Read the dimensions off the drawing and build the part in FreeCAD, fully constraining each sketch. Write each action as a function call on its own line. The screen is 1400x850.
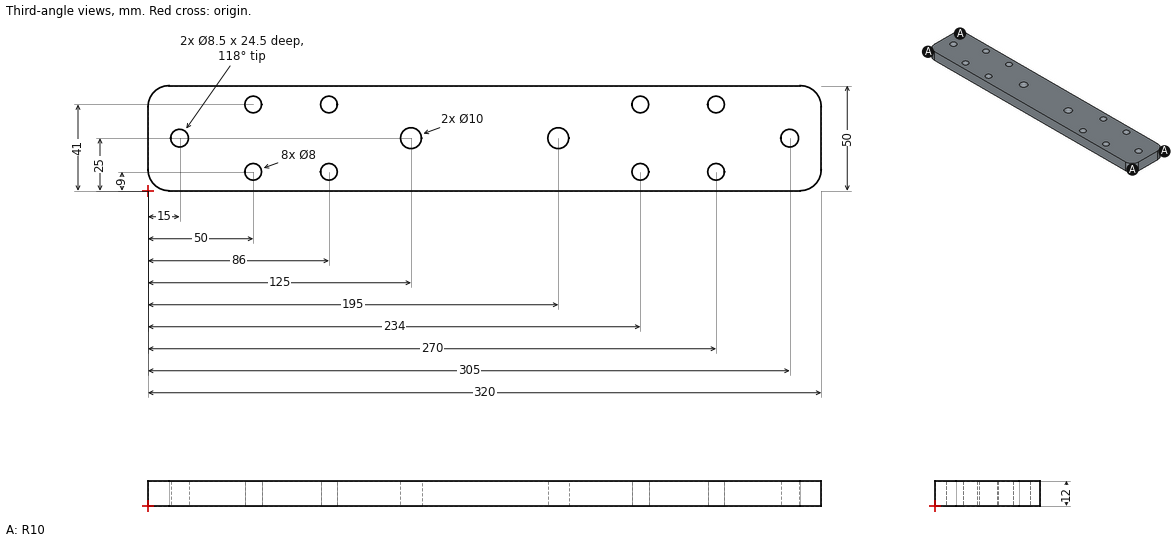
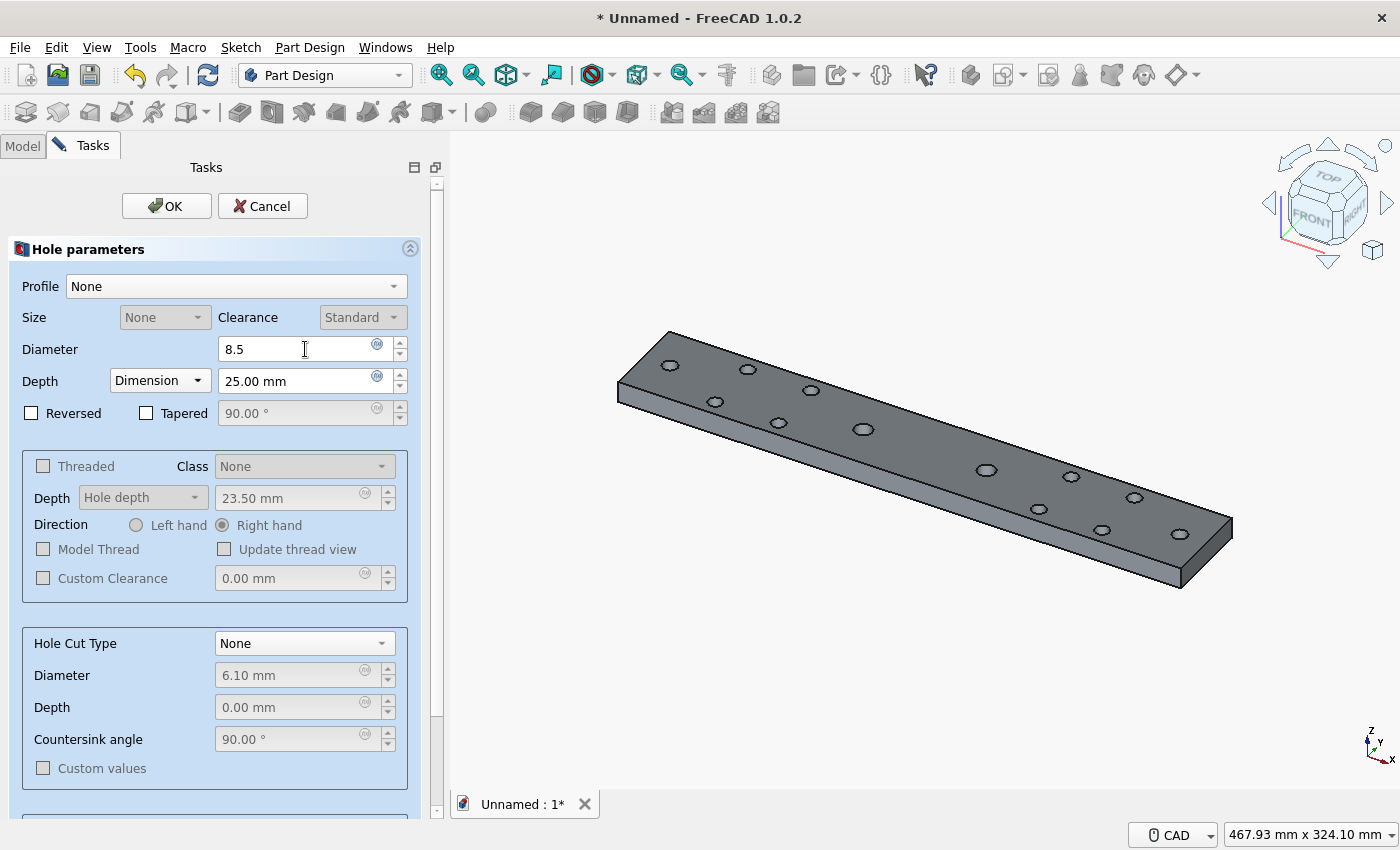
triple_click(305, 381)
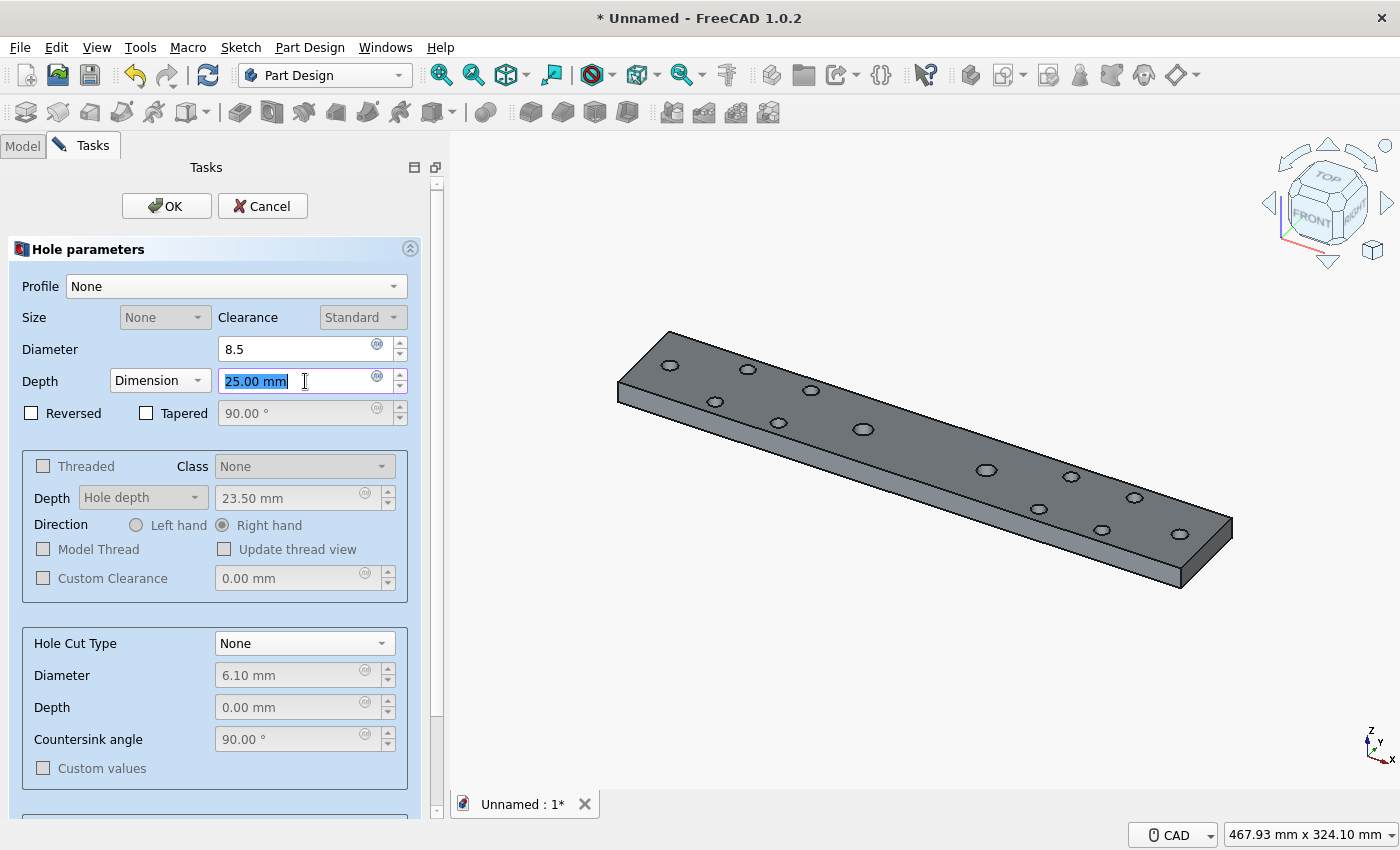
text(24.5)
key(Tab)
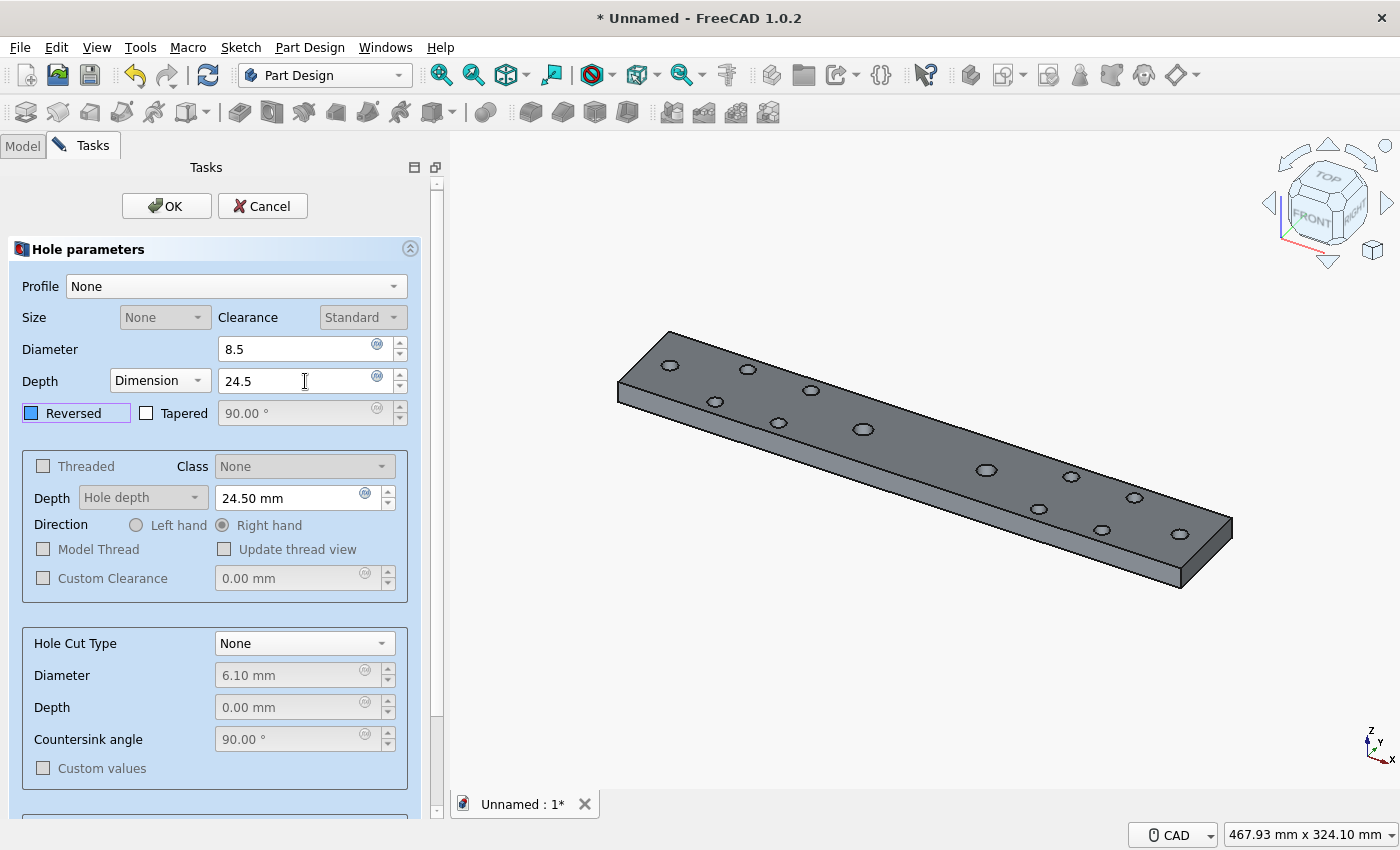
click(167, 206)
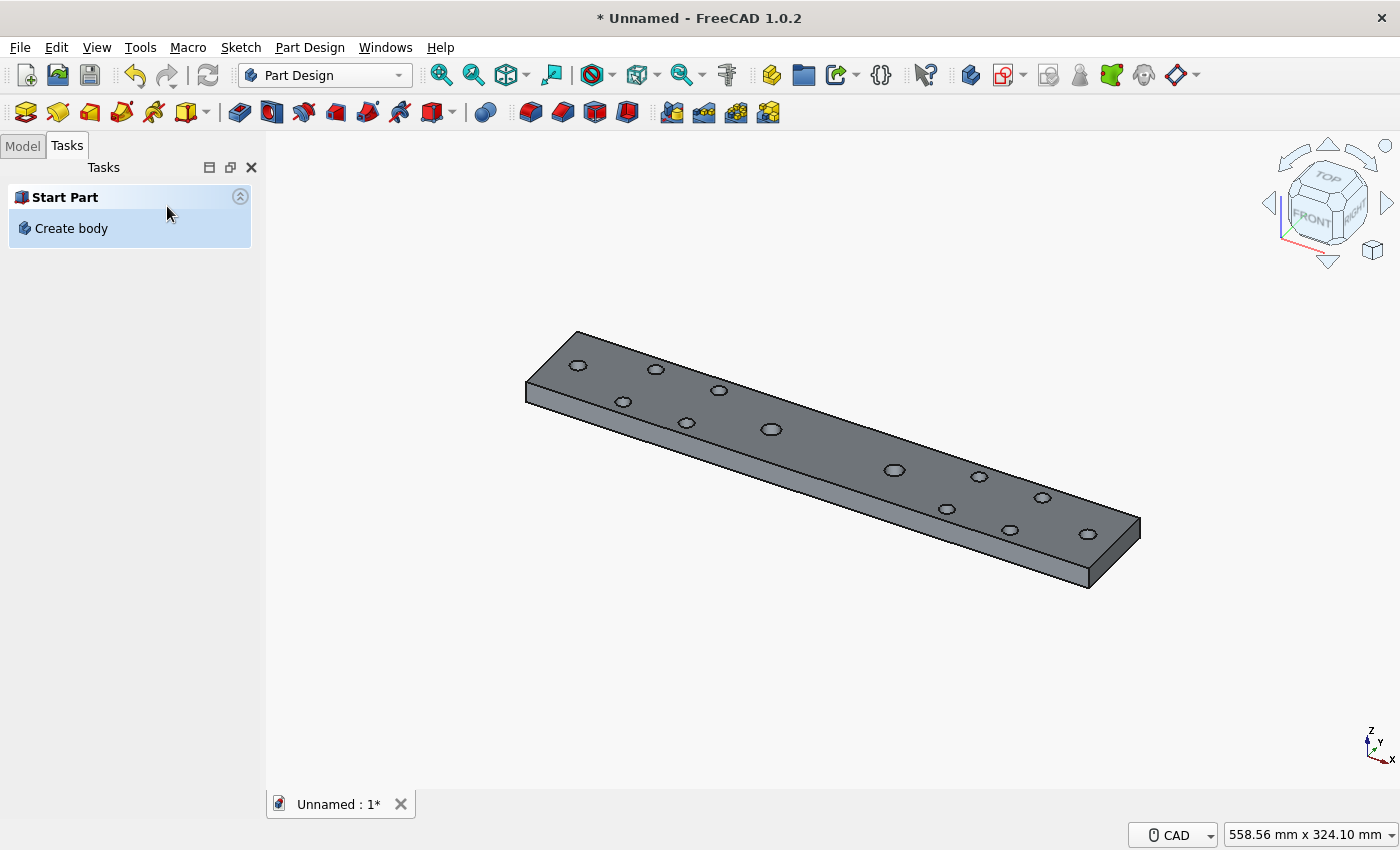
click(1089, 577)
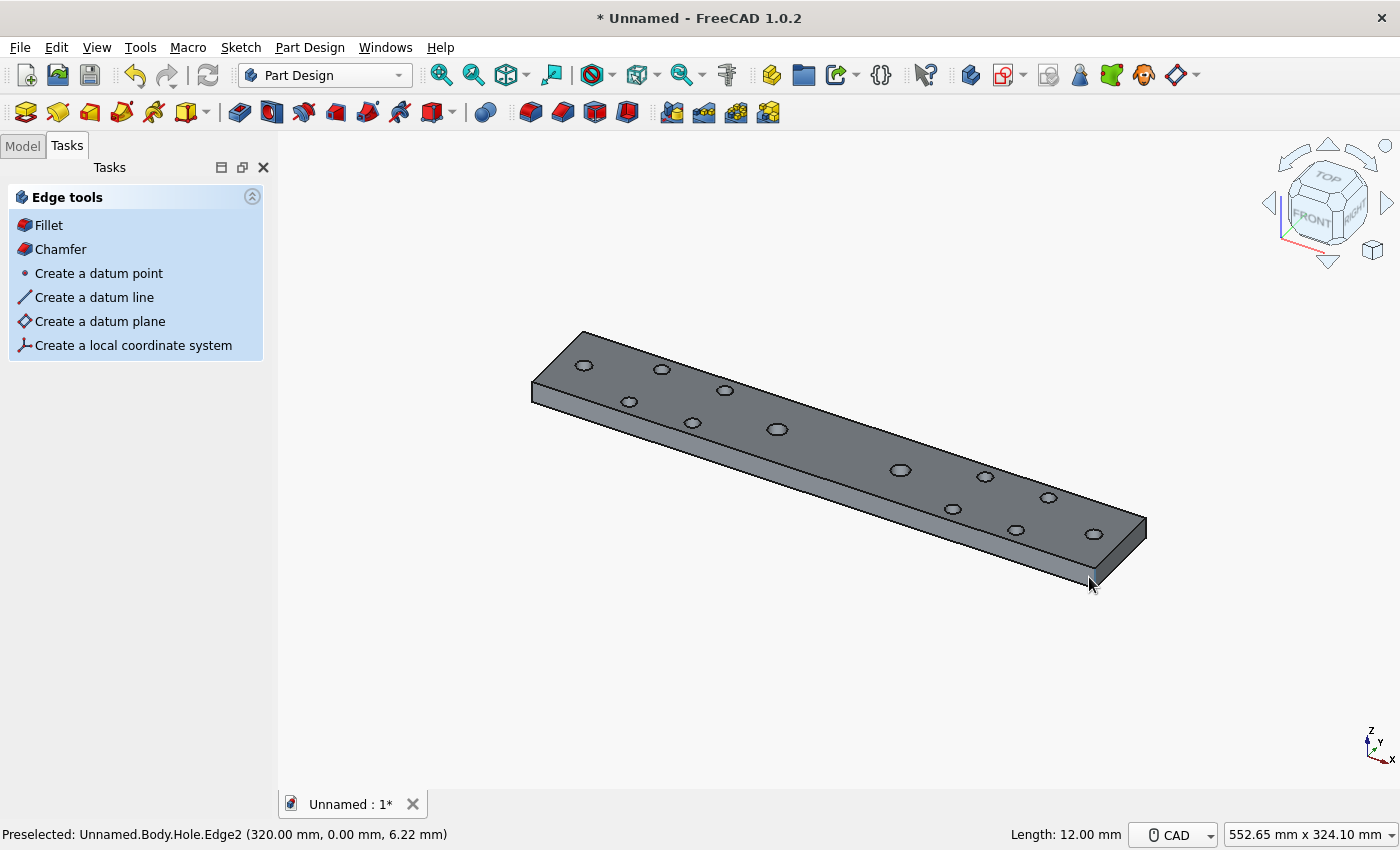
key(0)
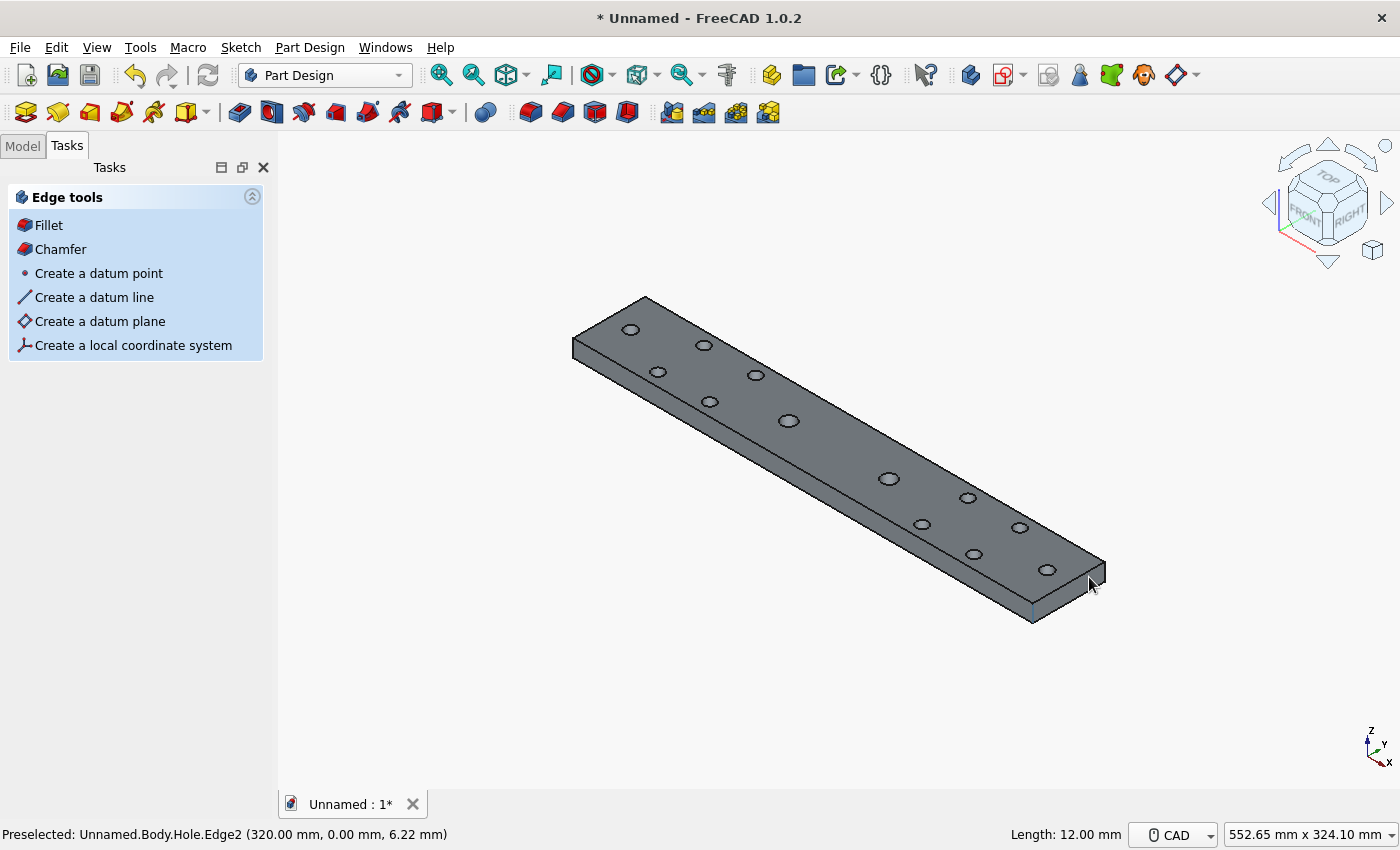
key(2)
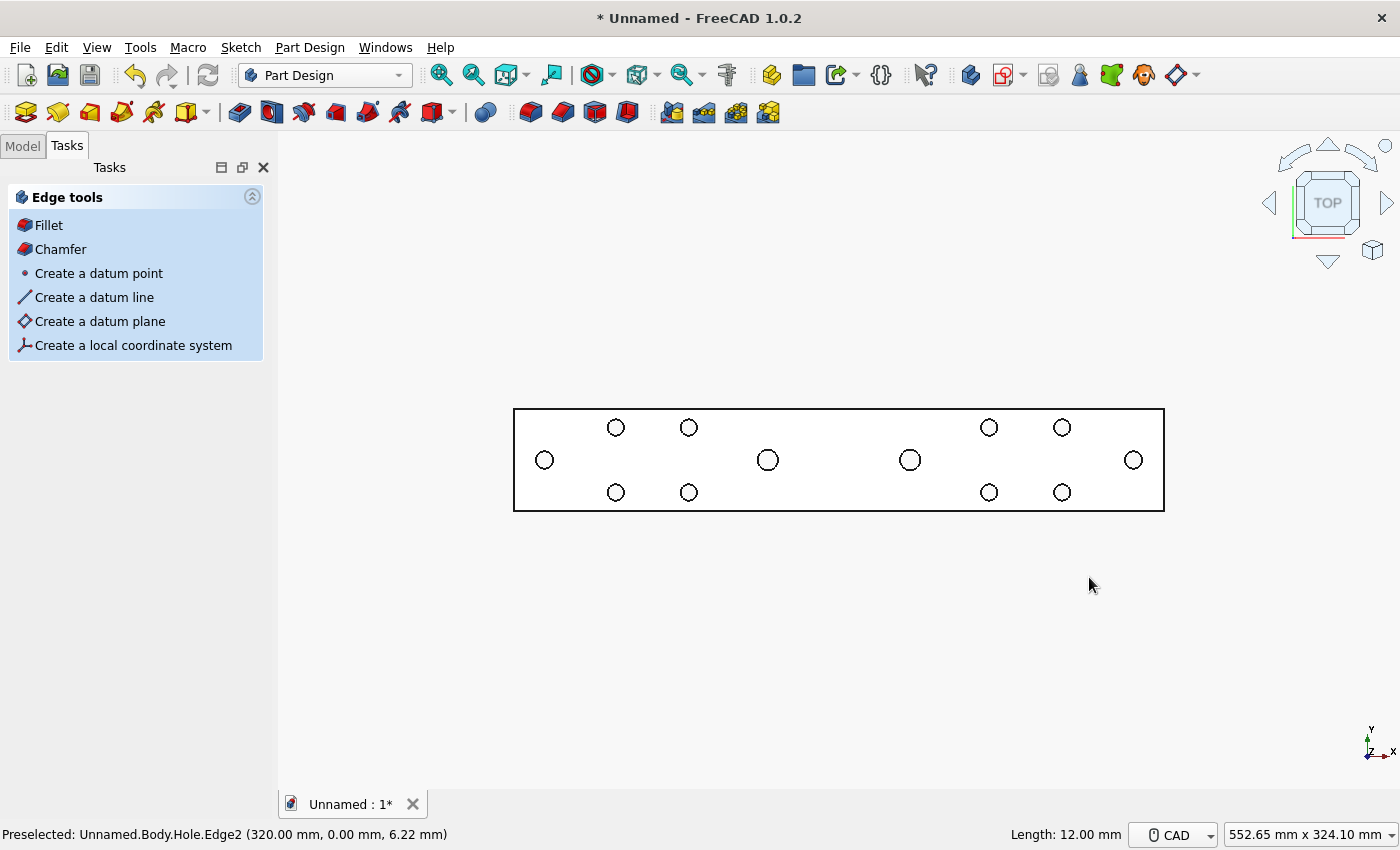
key(1)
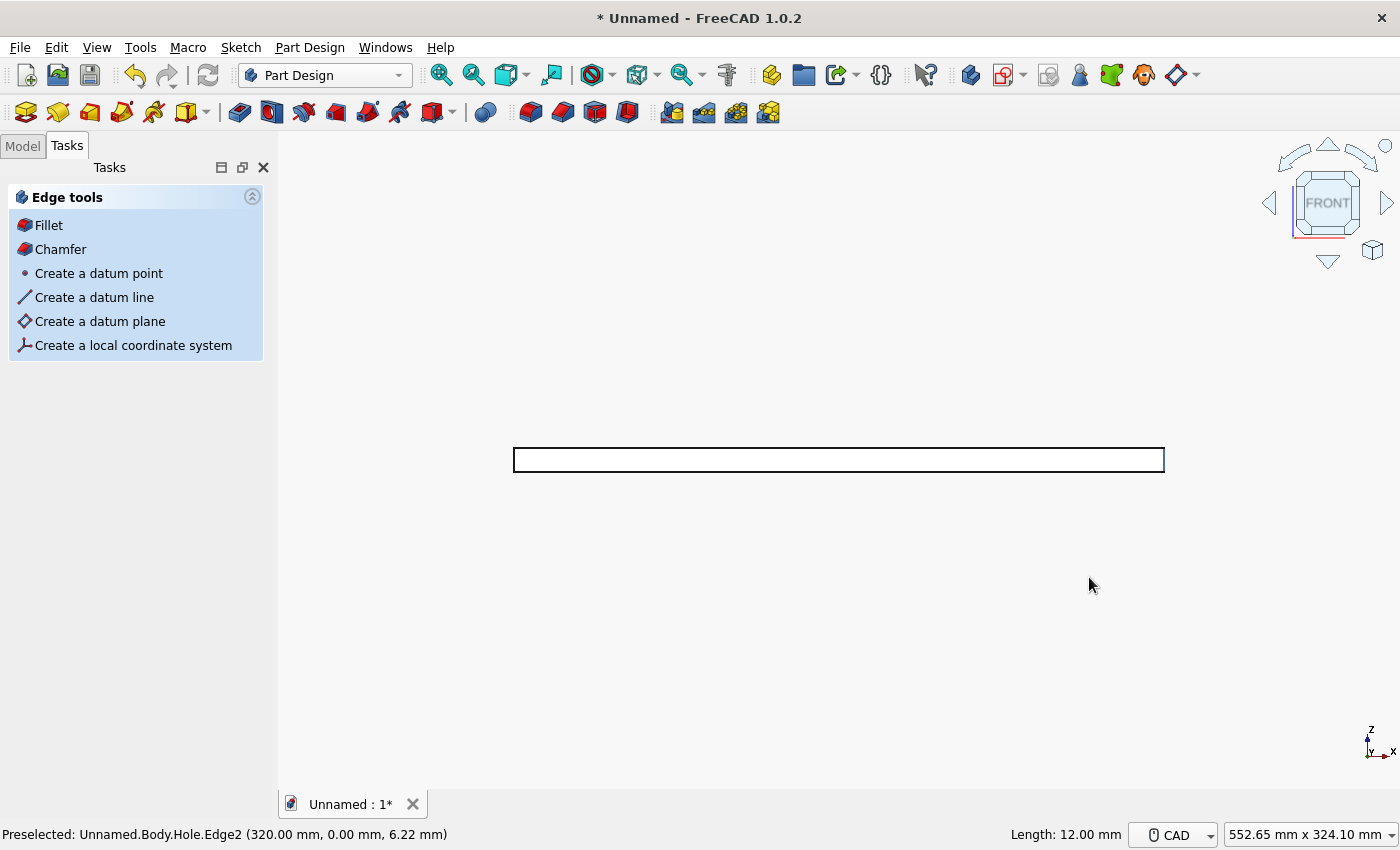
click(514, 459, ctrl)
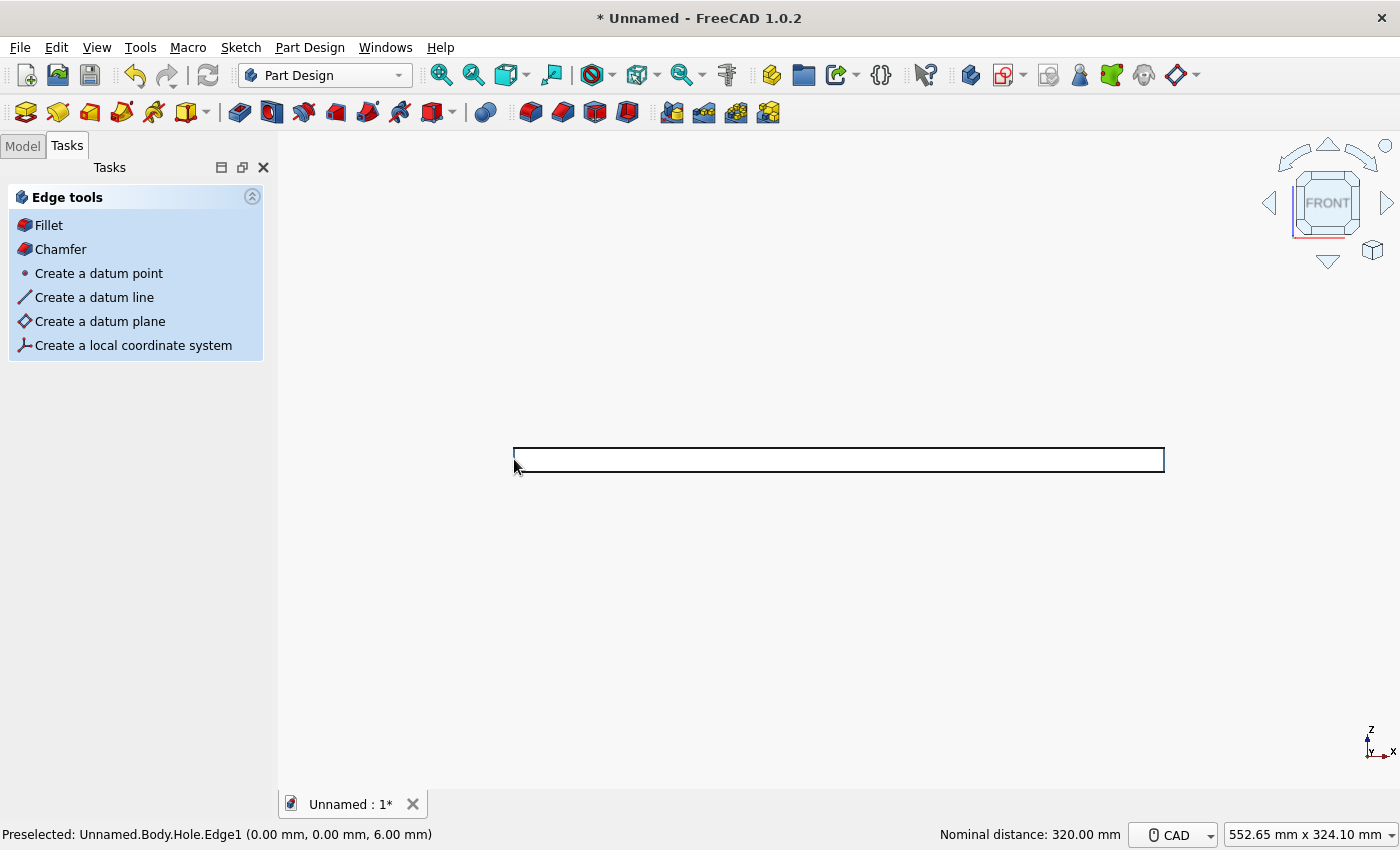
key(3)